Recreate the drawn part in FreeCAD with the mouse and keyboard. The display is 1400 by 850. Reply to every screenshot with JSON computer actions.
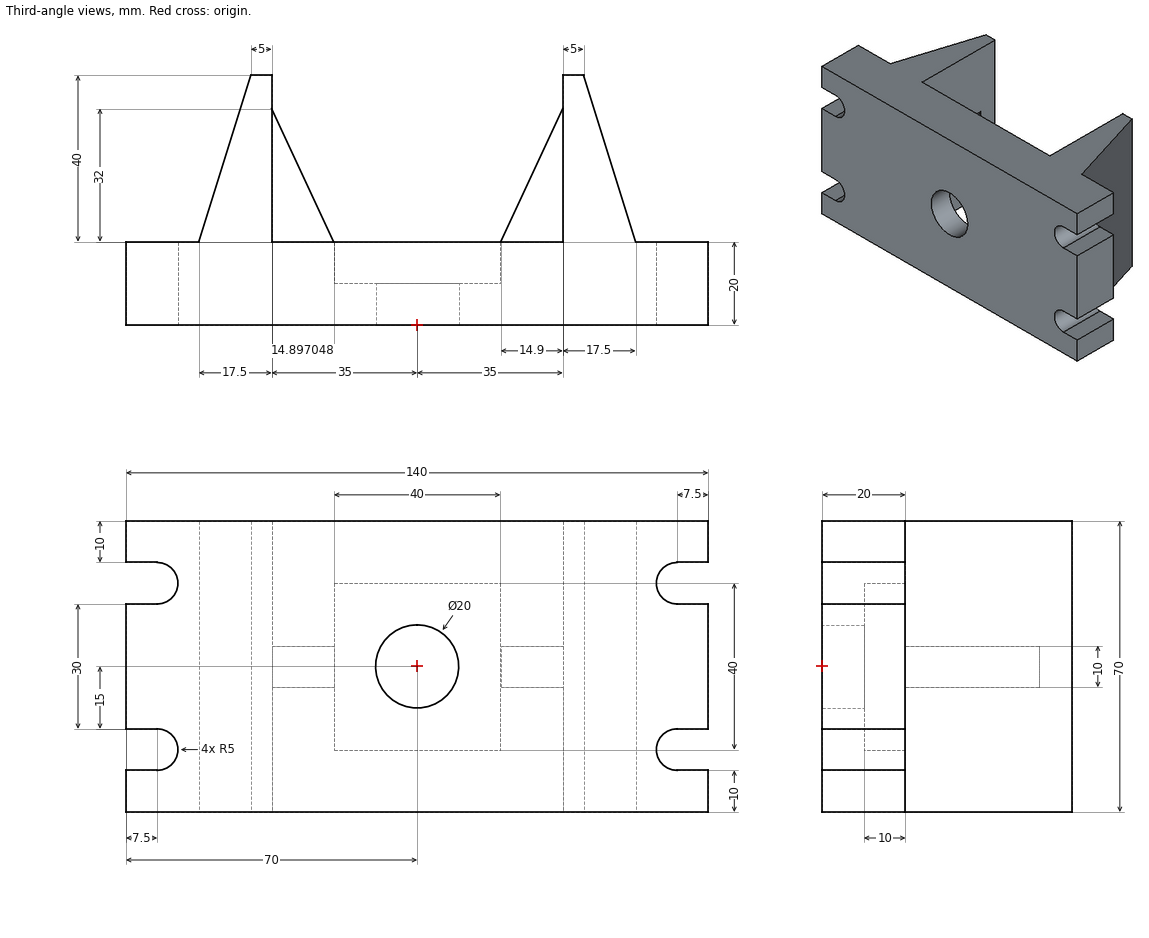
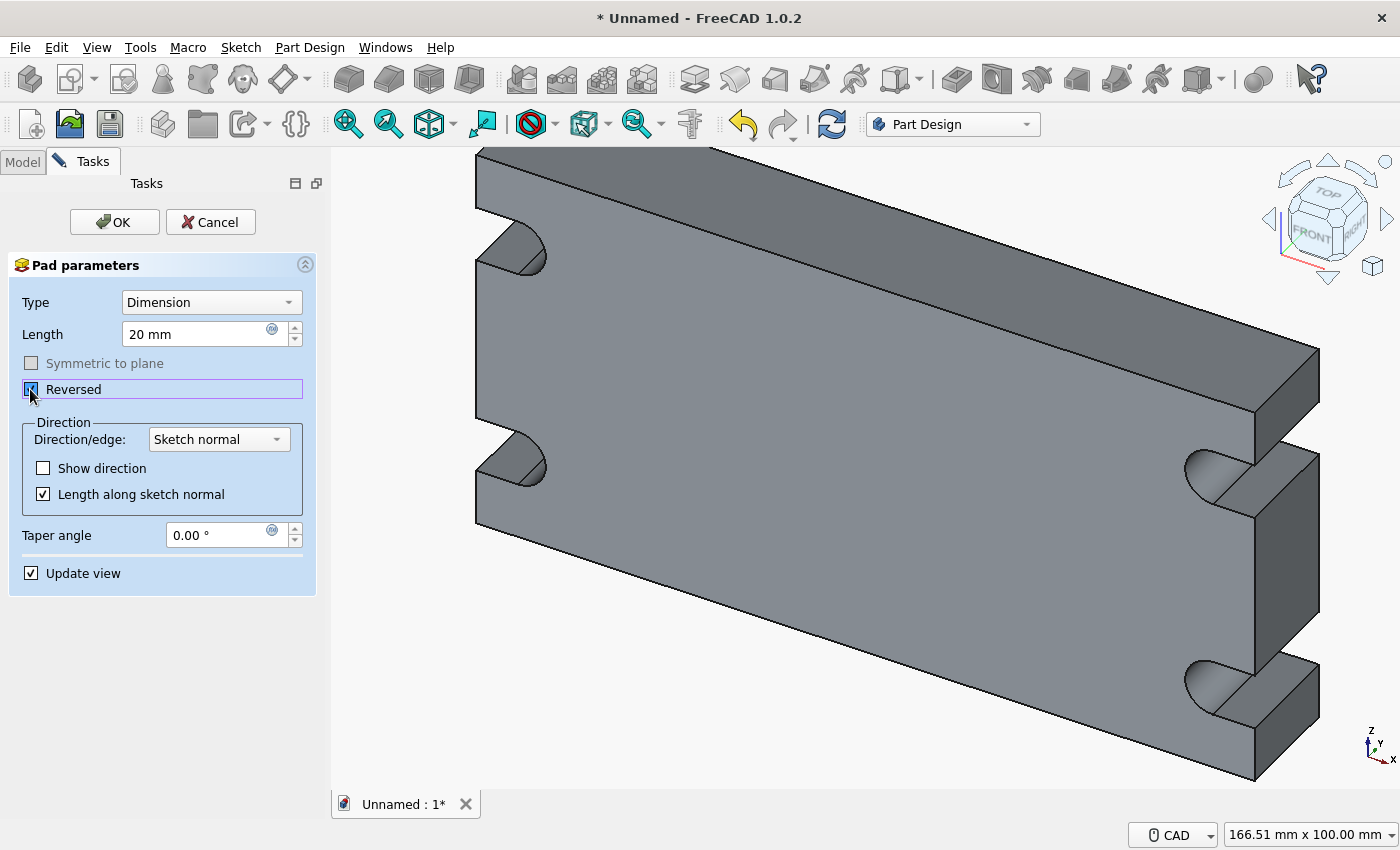
{"action": "left_click", "coordinate": [115, 222]}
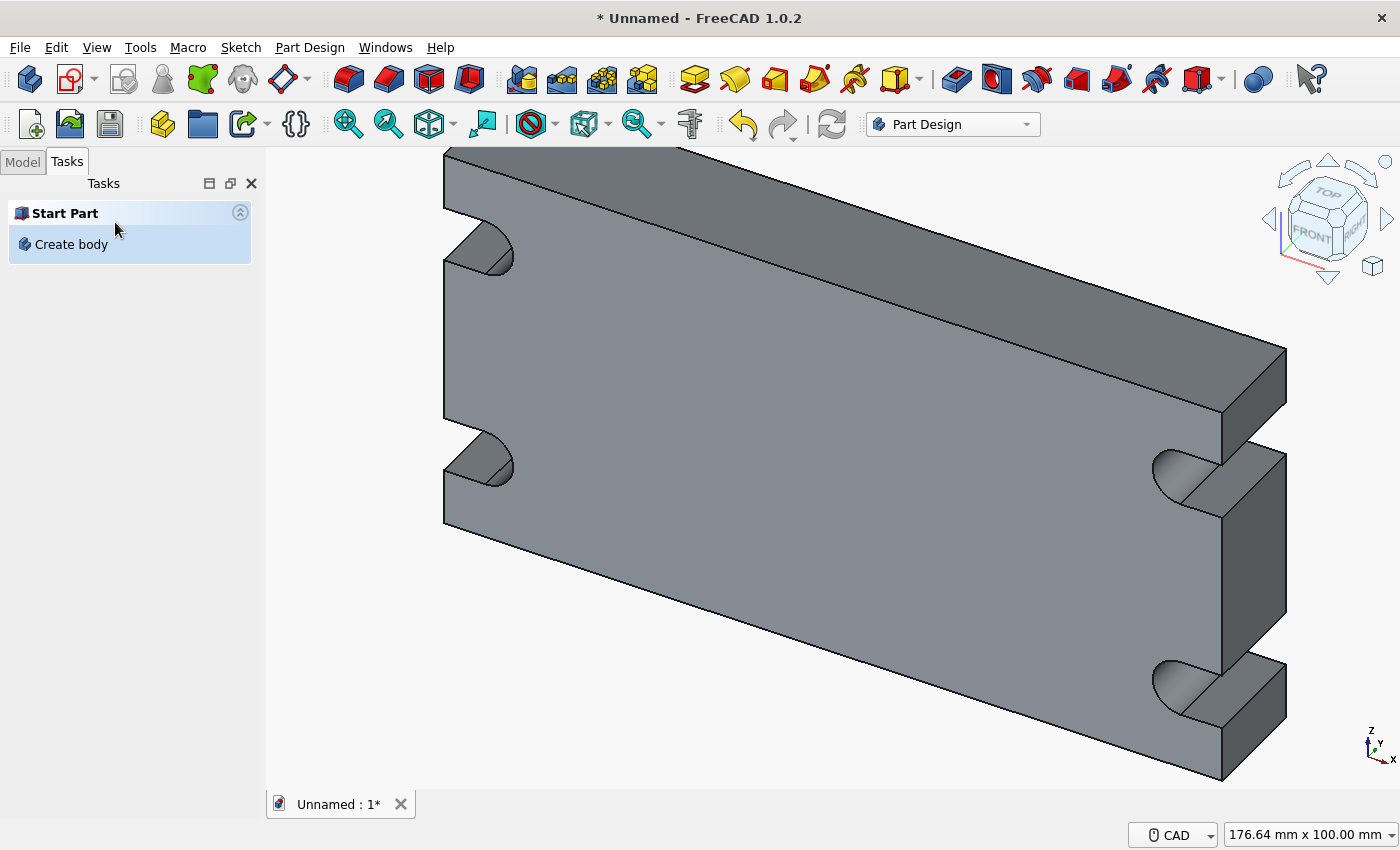
{"action": "left_click", "coordinate": [350, 124]}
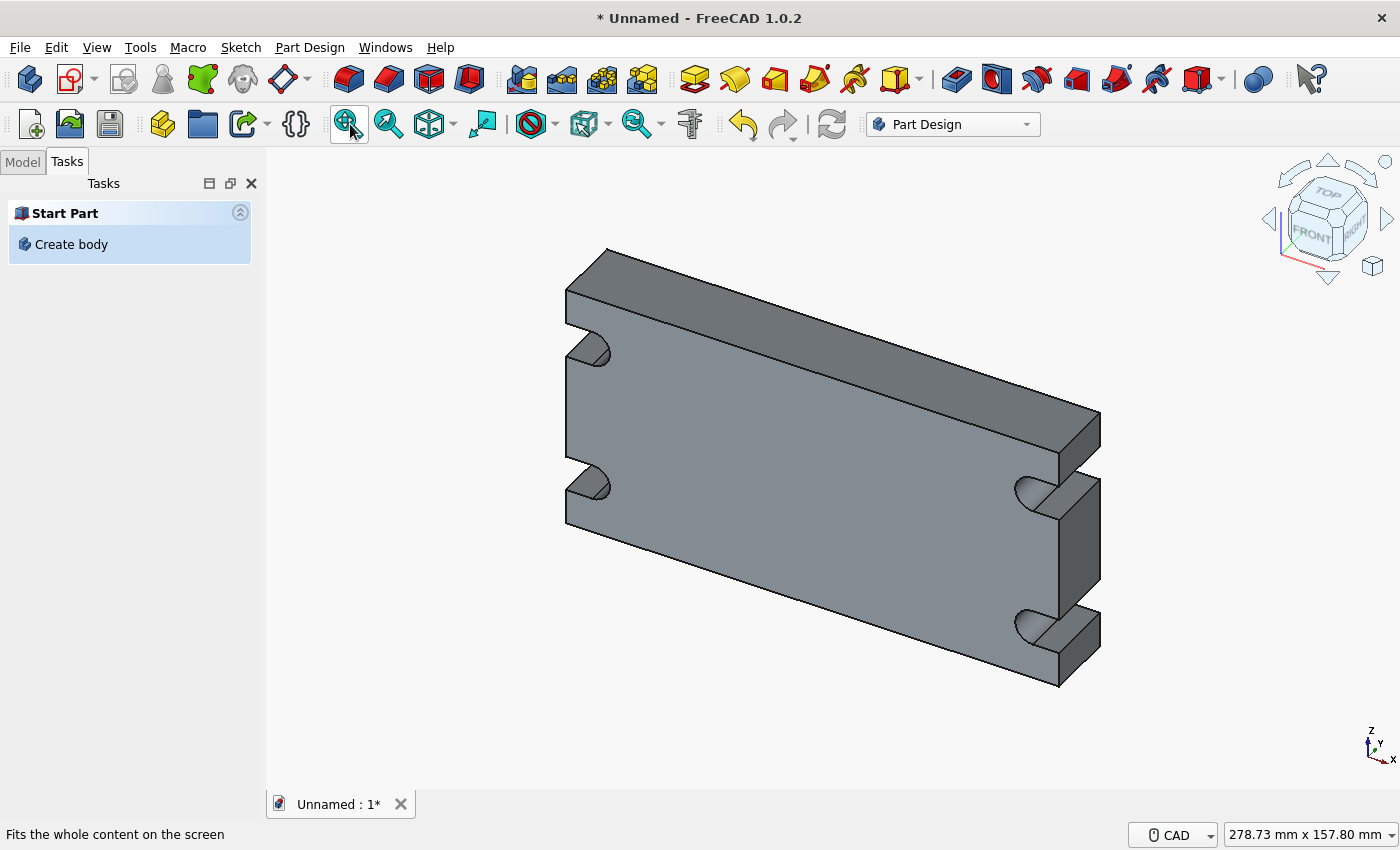
{"action": "key", "text": "4"}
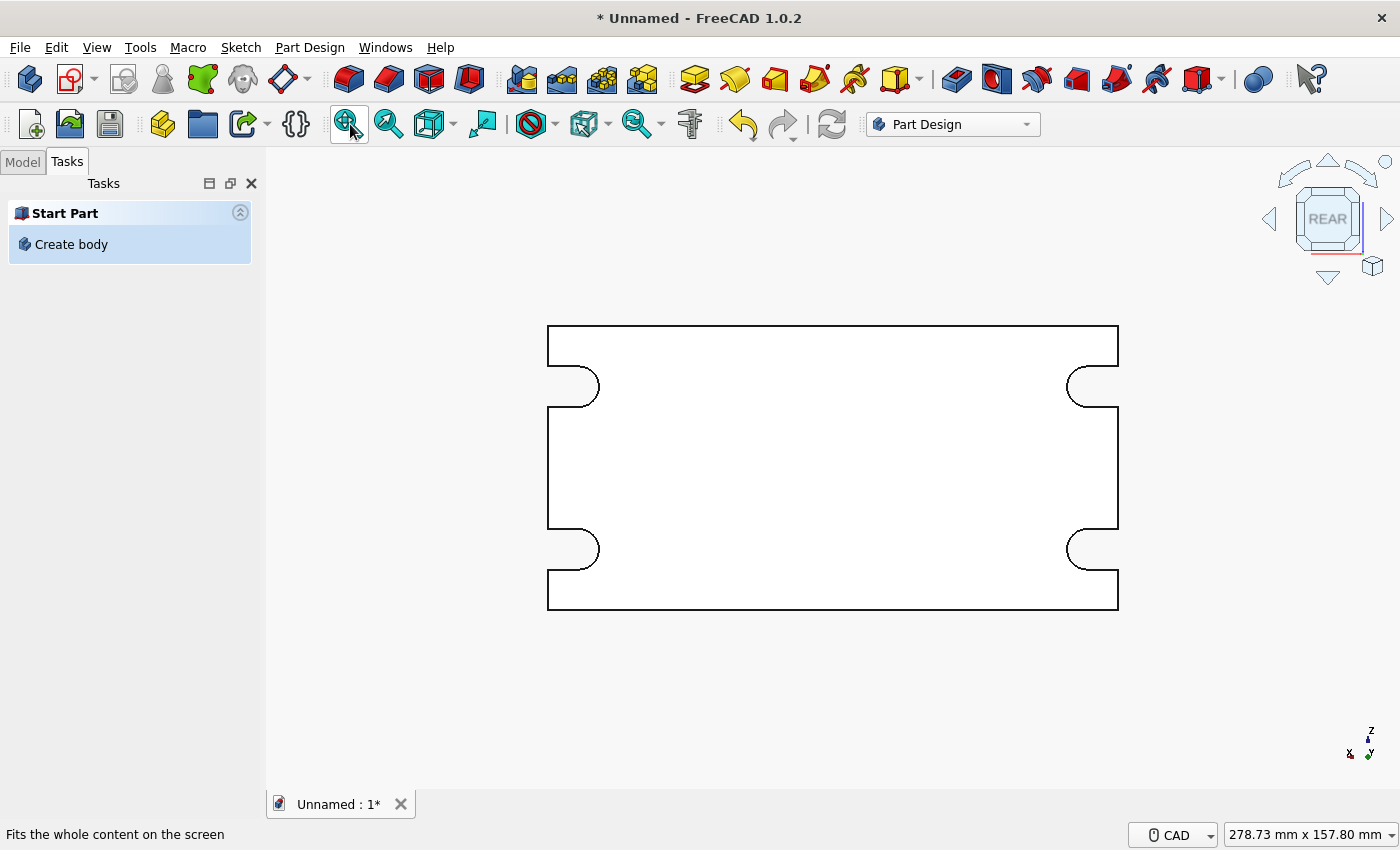
{"action": "left_click", "coordinate": [752, 467]}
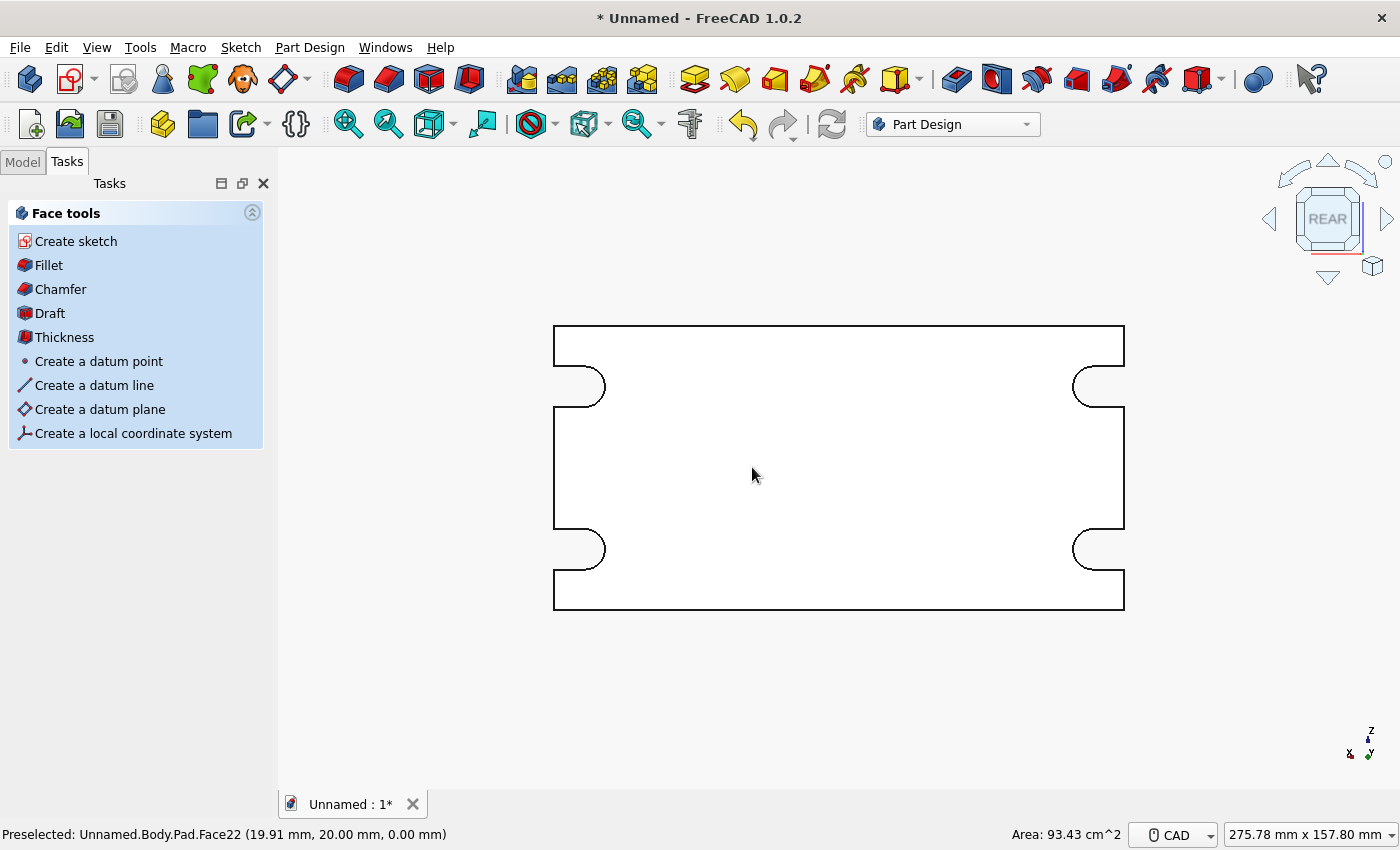
{"action": "left_click", "coordinate": [70, 80]}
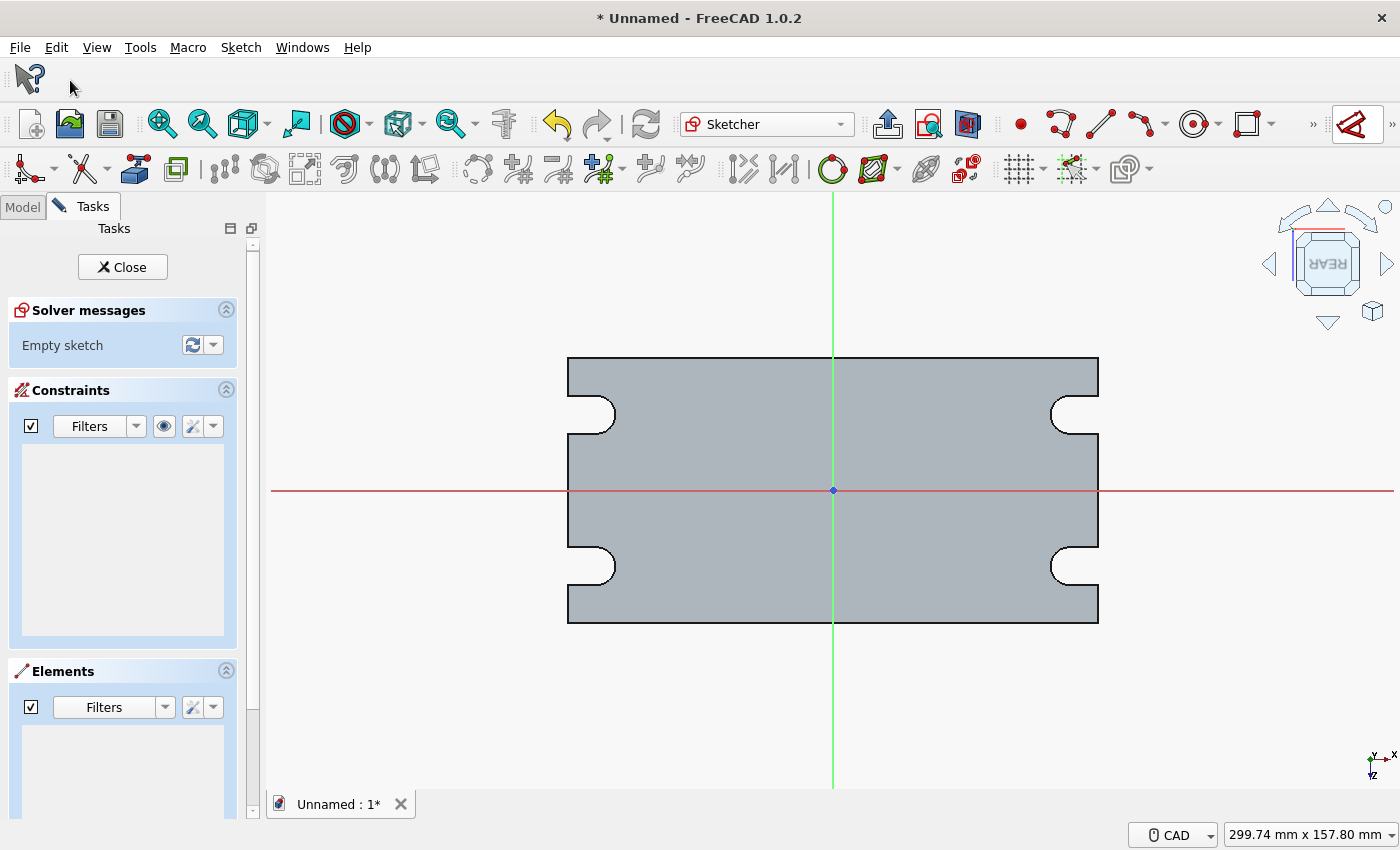
{"action": "scroll", "coordinate": [850, 491], "scroll_direction": "up", "scroll_amount": 8}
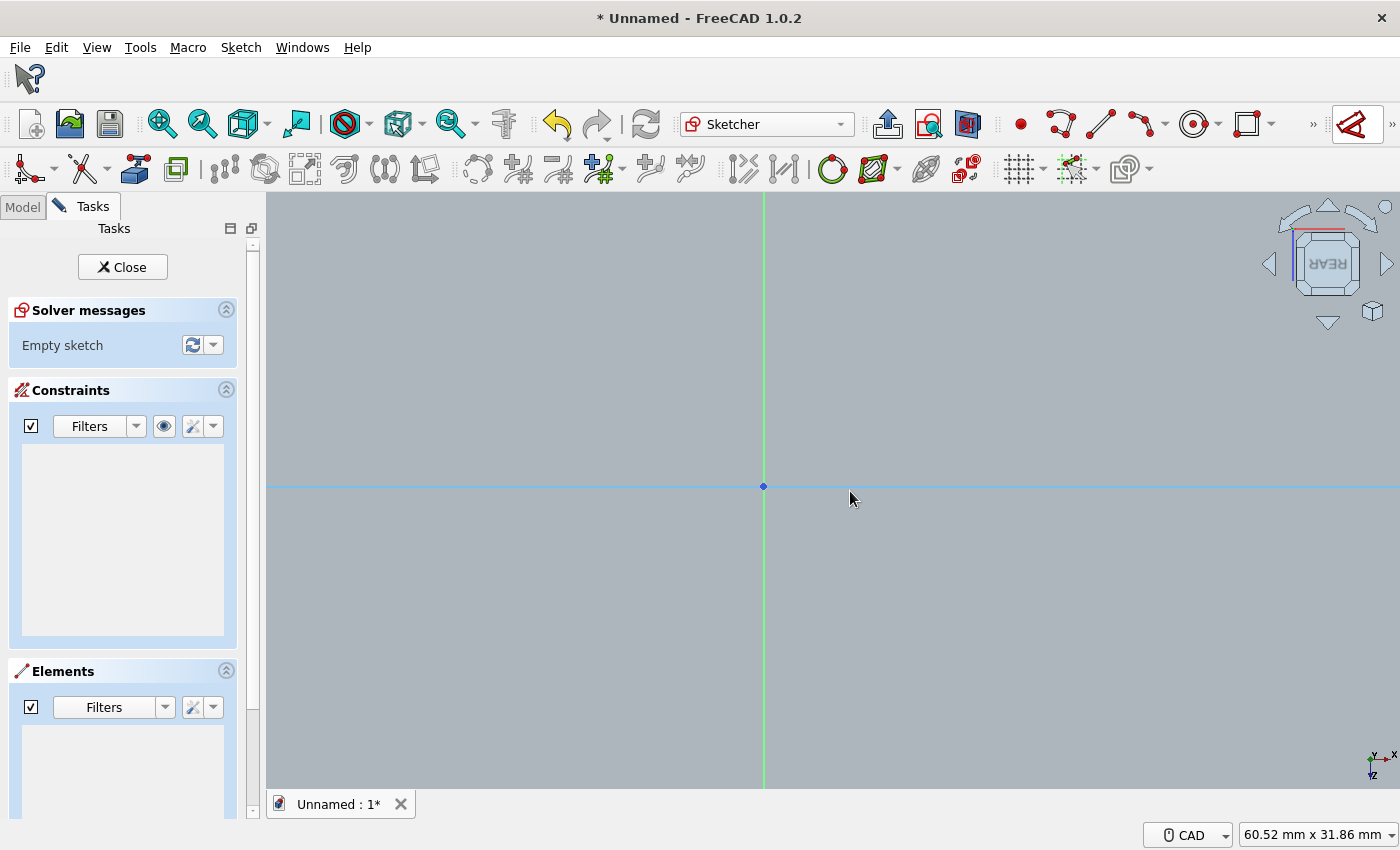
{"action": "left_click", "coordinate": [1194, 124]}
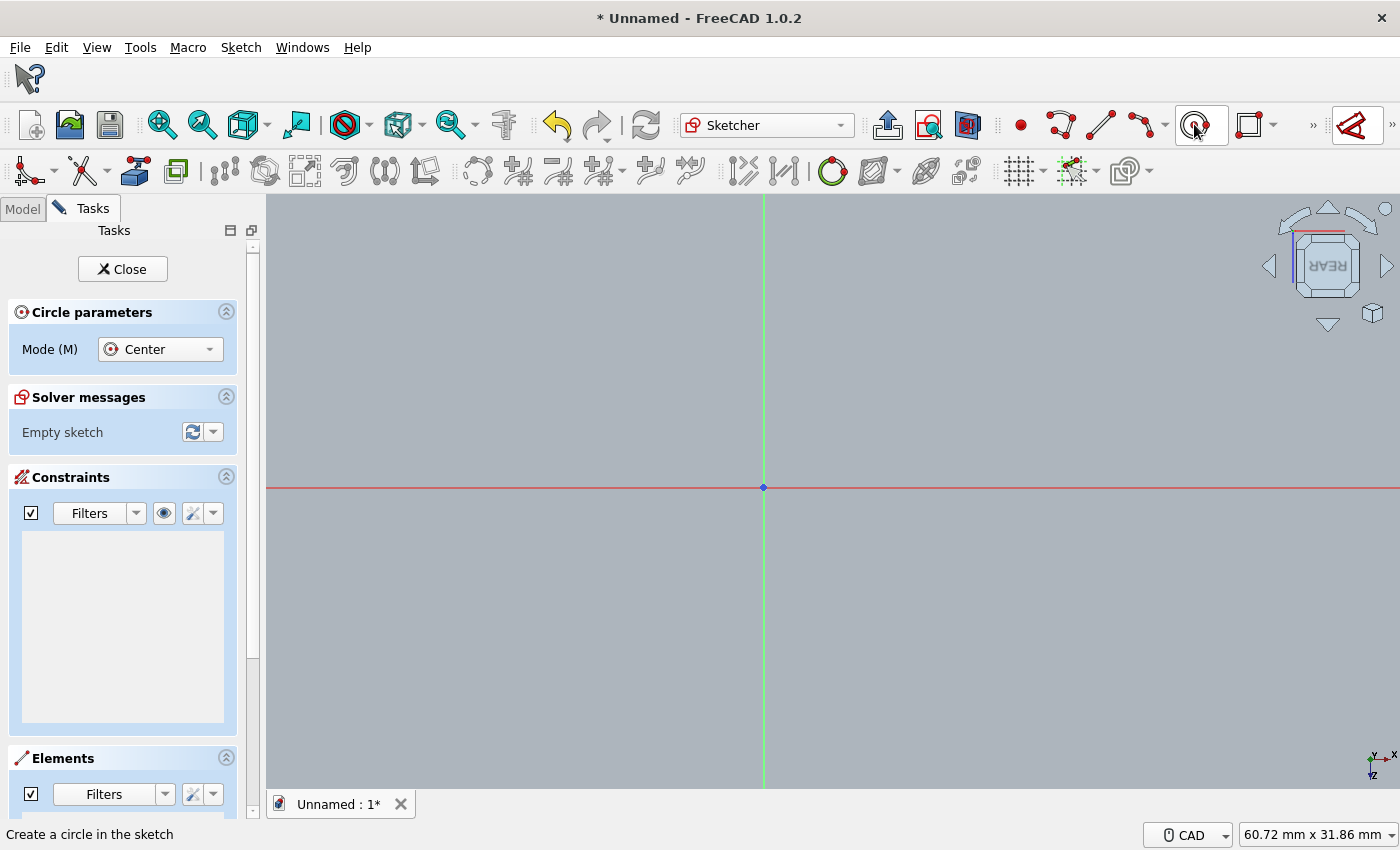
{"action": "left_click", "coordinate": [764, 488]}
{"action": "mouse_move", "coordinate": [896, 355]}